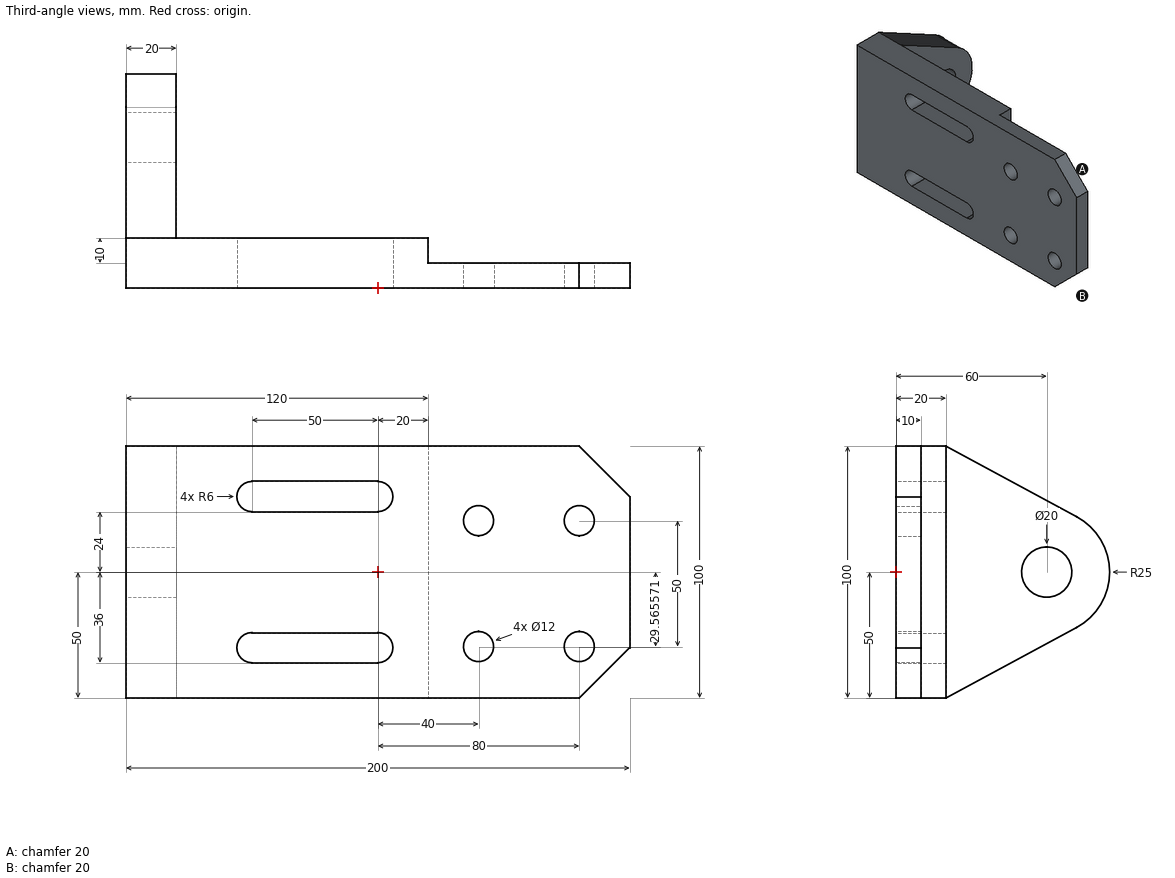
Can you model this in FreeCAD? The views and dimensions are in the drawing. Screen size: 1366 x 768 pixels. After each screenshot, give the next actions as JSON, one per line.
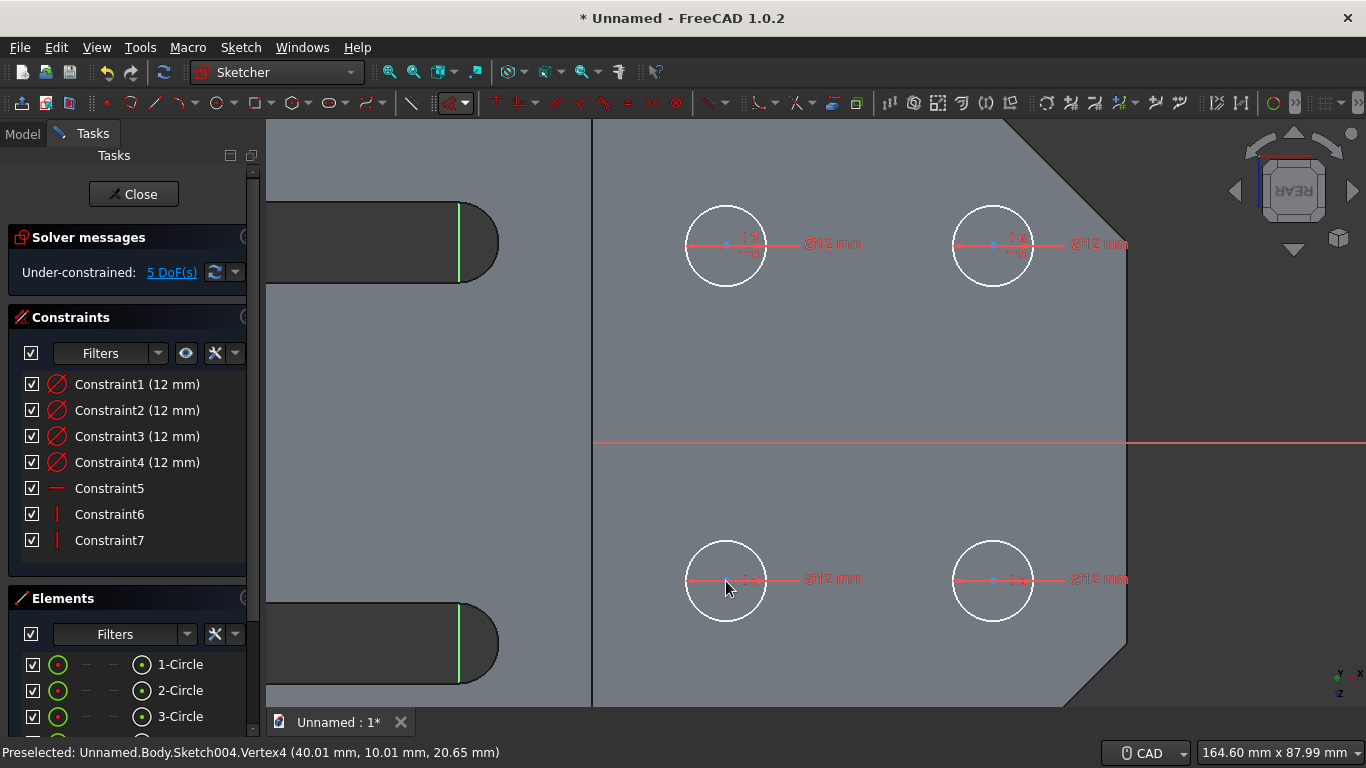
{"action": "left_click", "coordinate": [993, 581]}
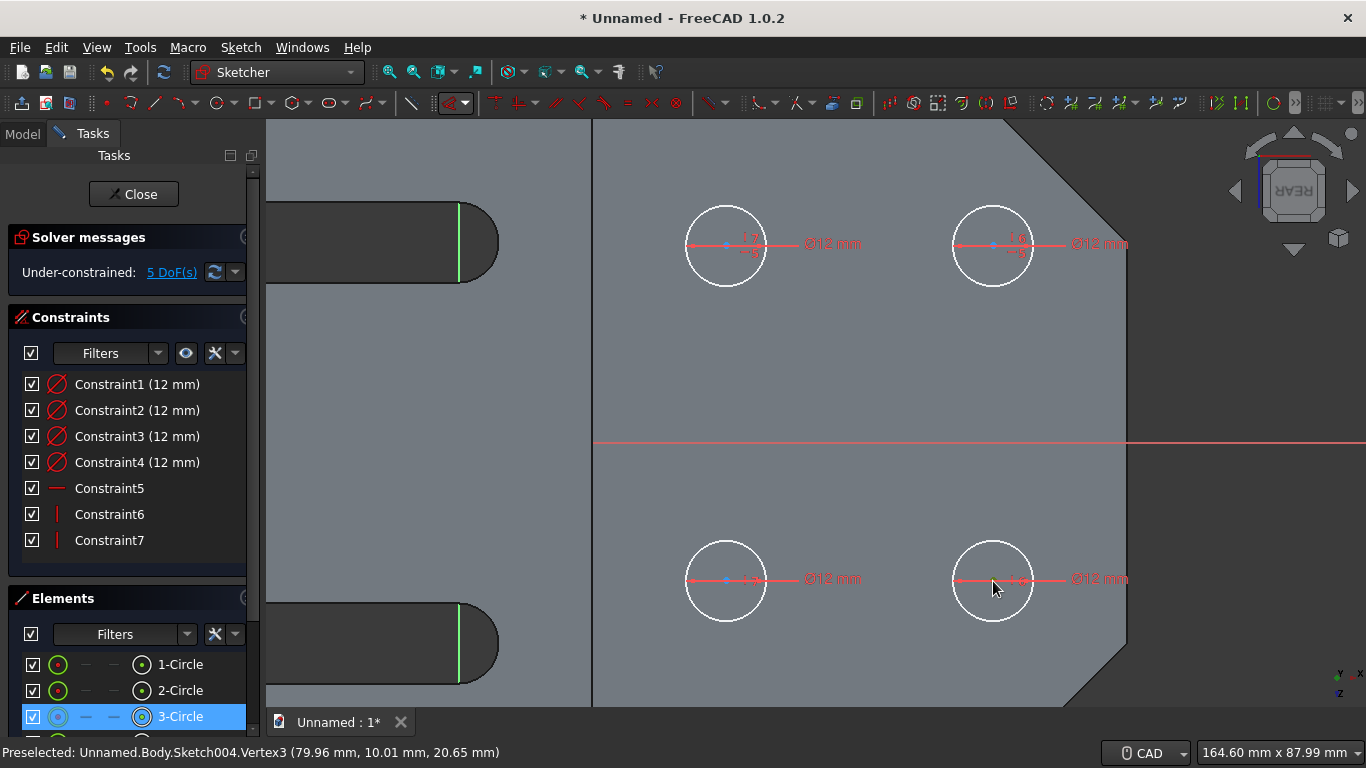
{"action": "left_click", "coordinate": [726, 581]}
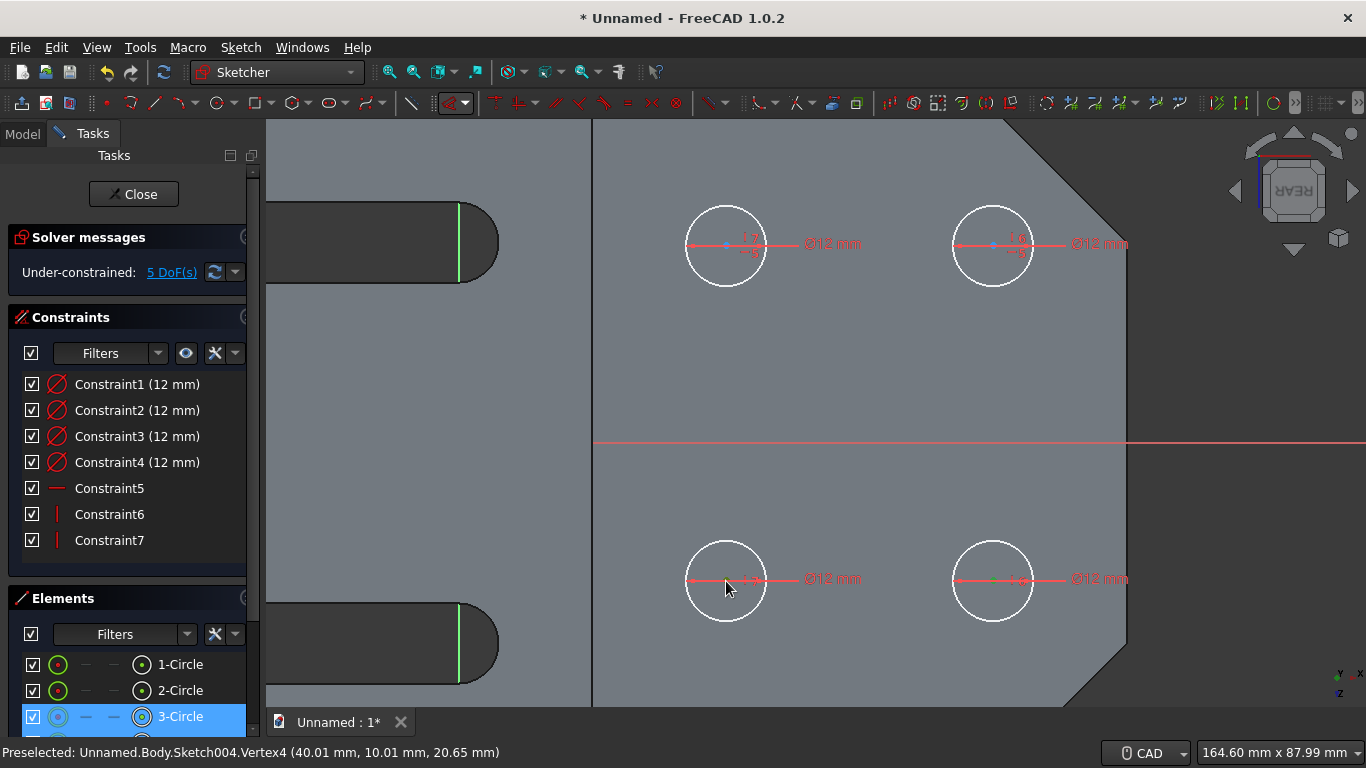
{"action": "left_click", "coordinate": [538, 104]}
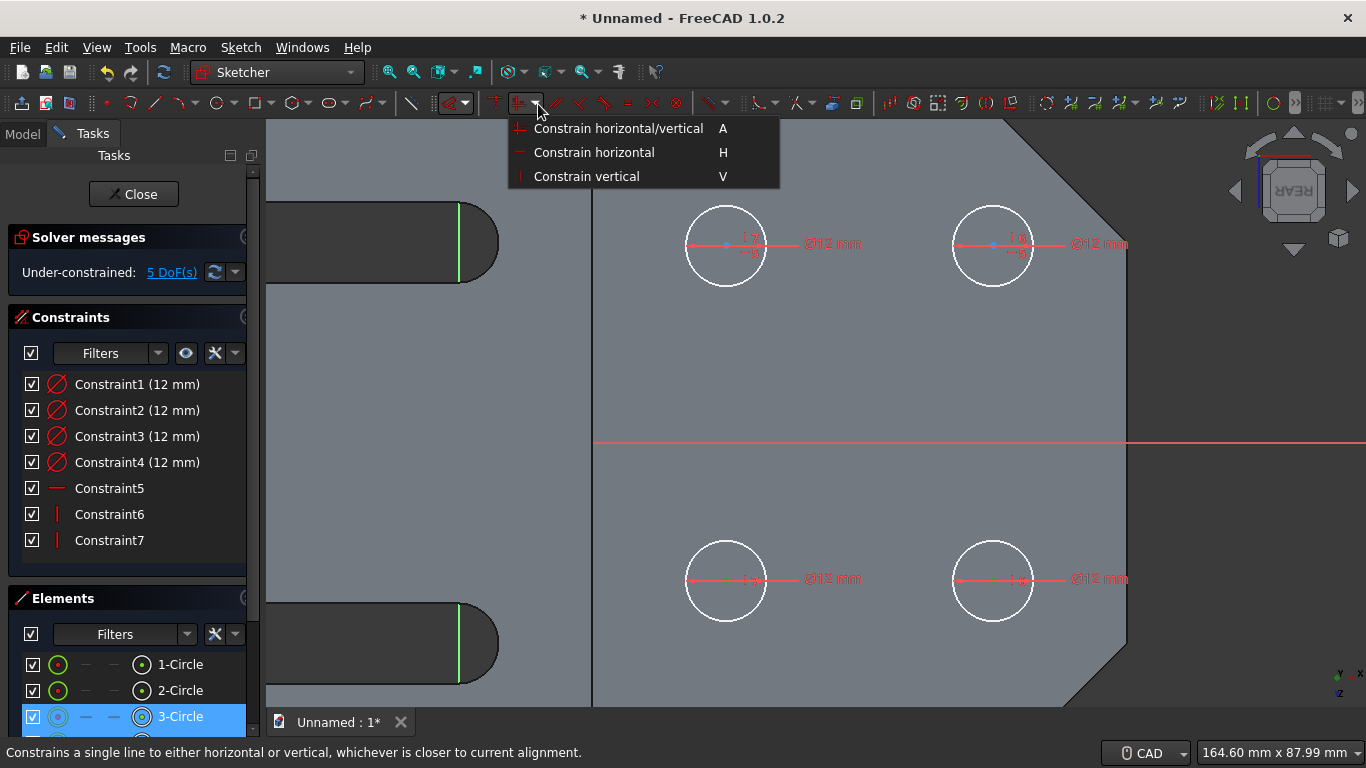
{"action": "left_click", "coordinate": [644, 152]}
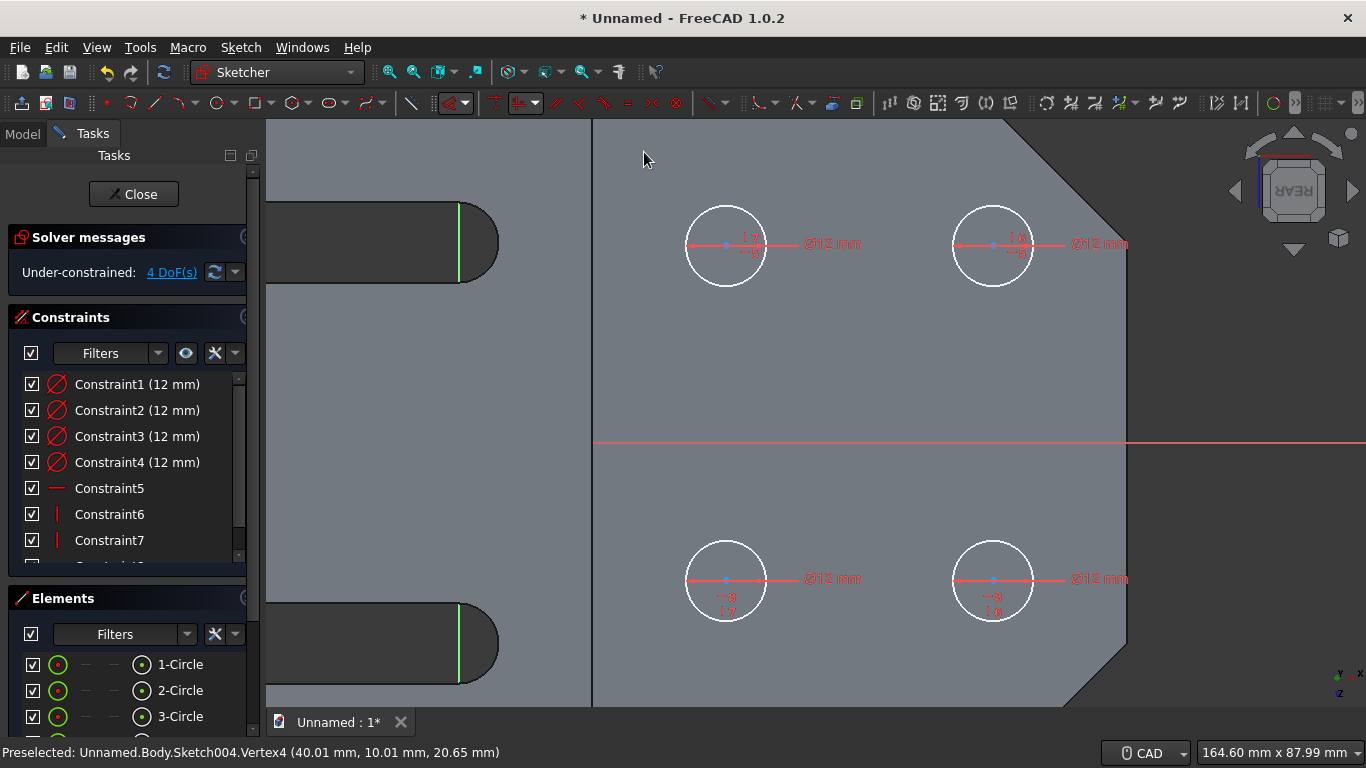
{"action": "left_click", "coordinate": [726, 246]}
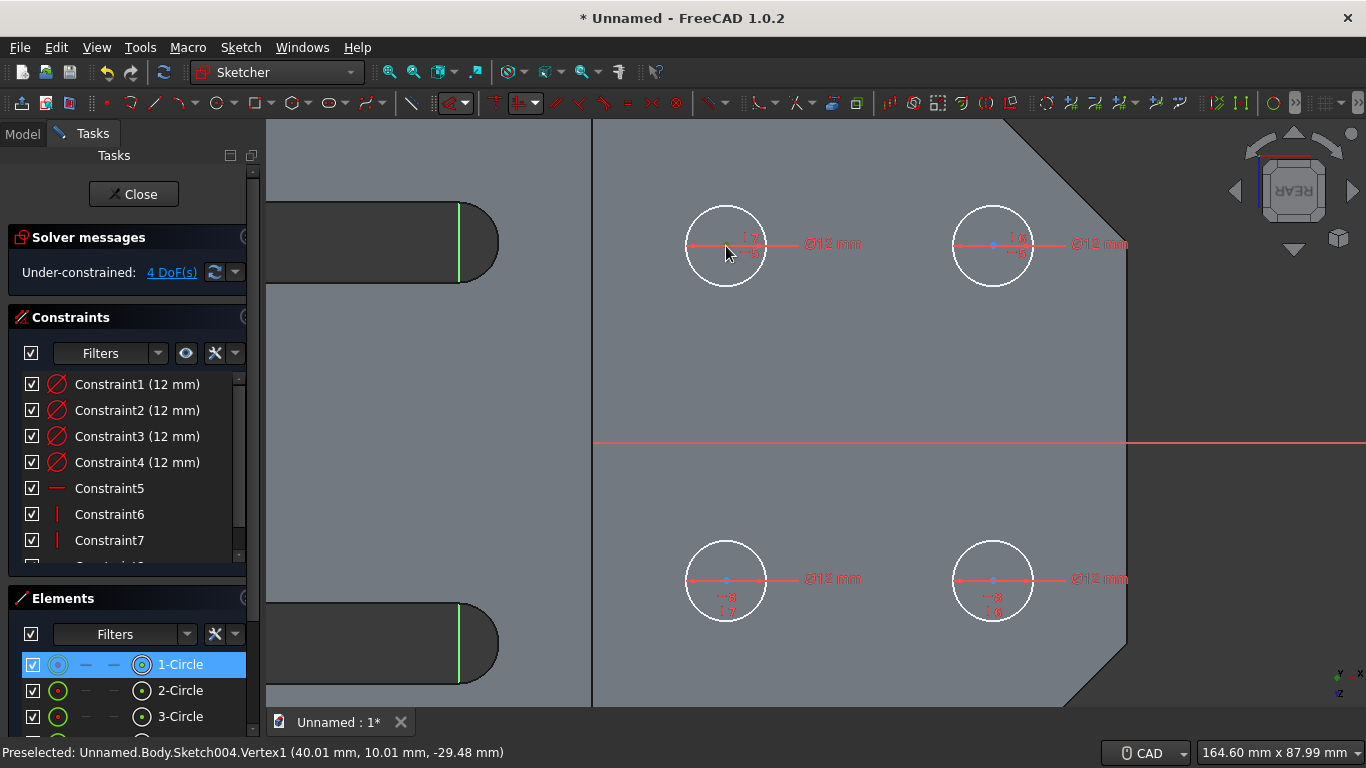
{"action": "left_click", "coordinate": [468, 104]}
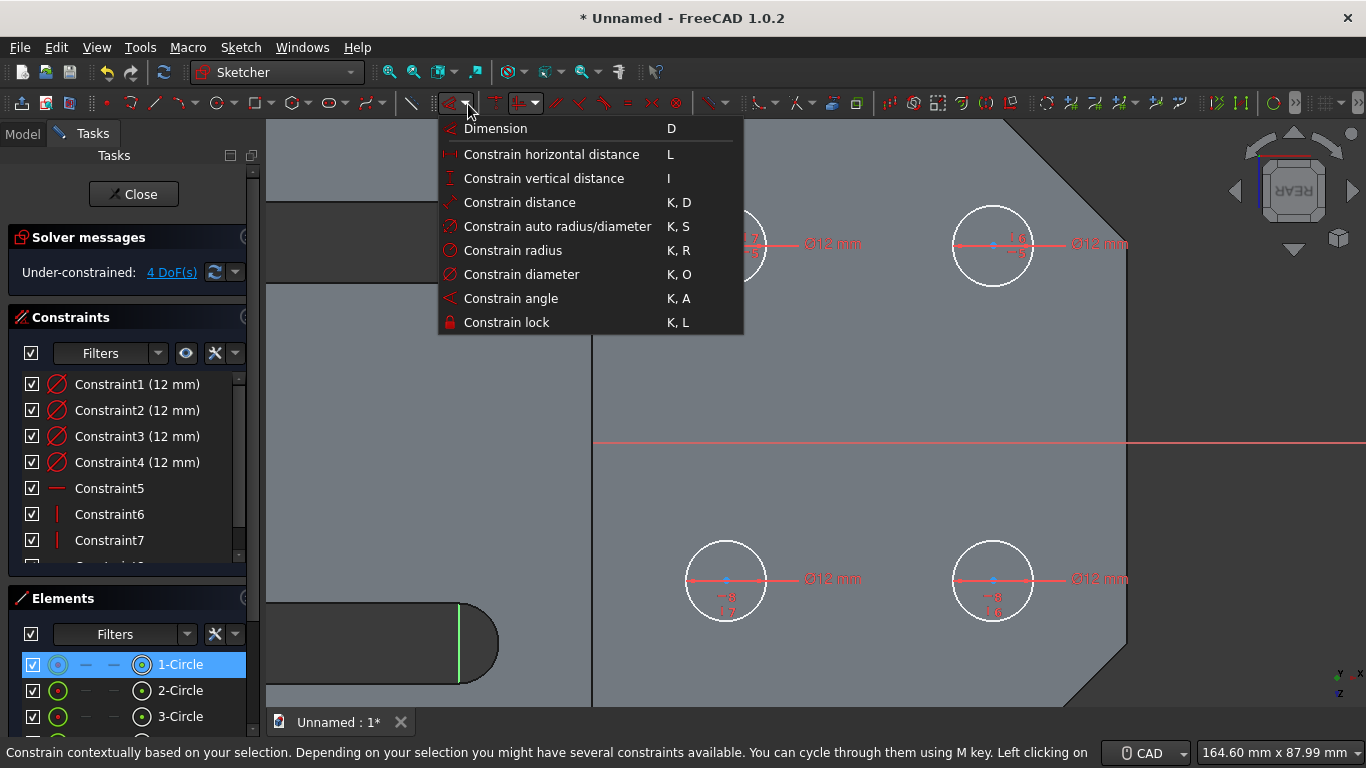
{"action": "left_click", "coordinate": [591, 154]}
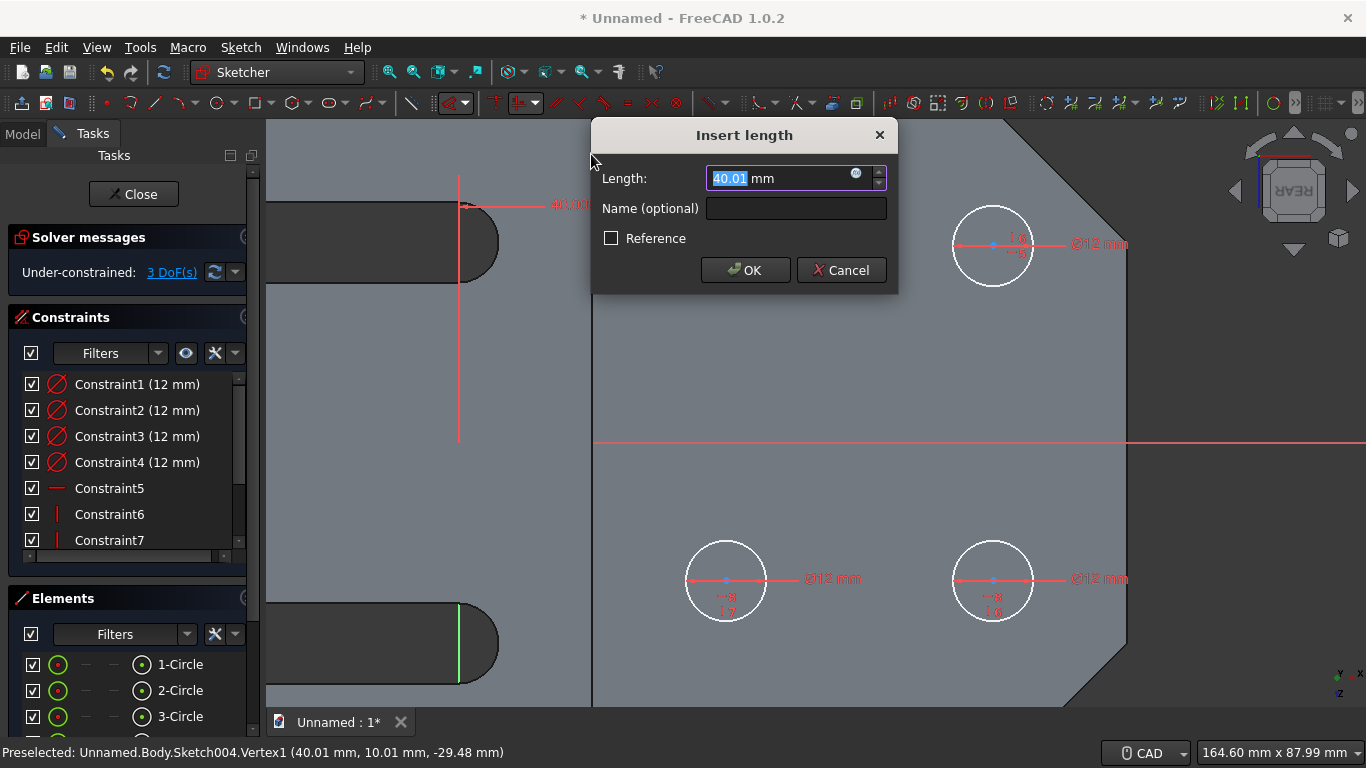
{"action": "type", "text": "40"}
{"action": "key", "text": "Return"}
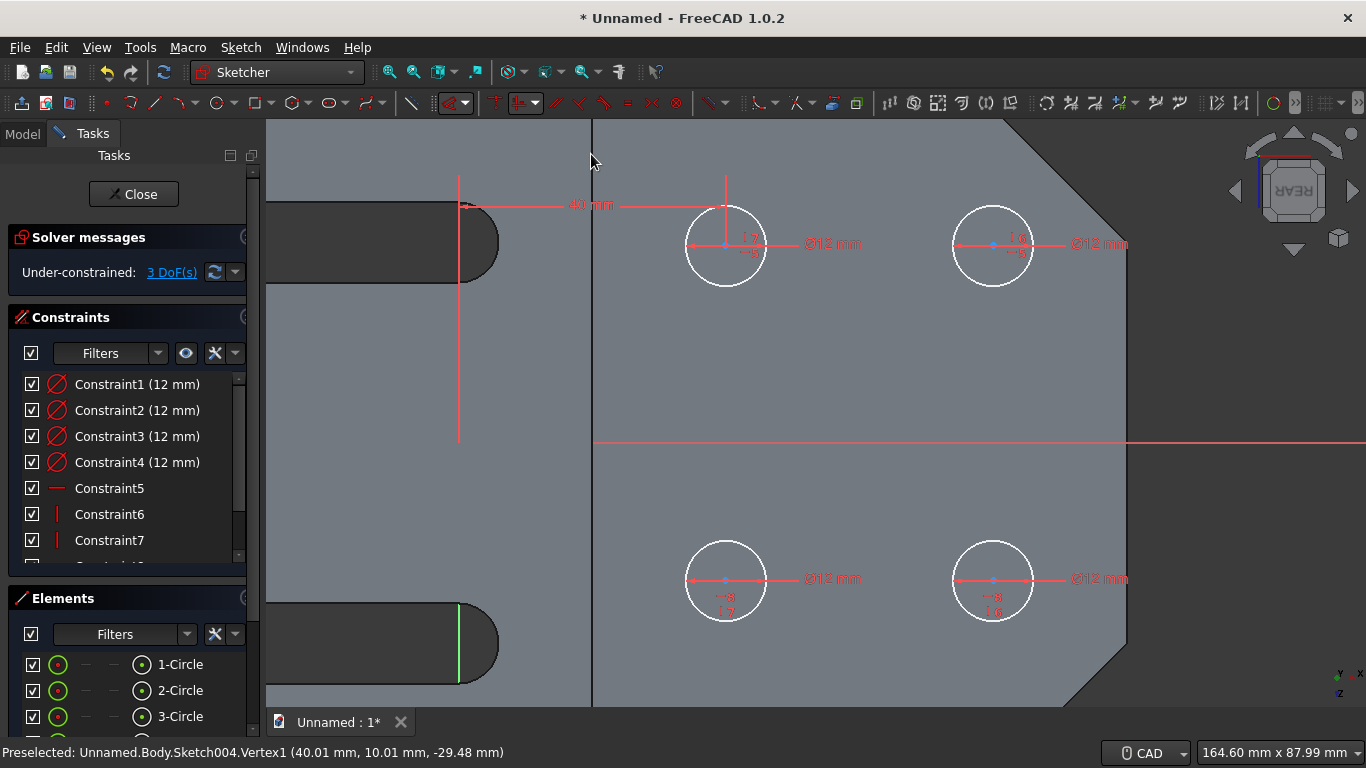
{"action": "left_click", "coordinate": [993, 246]}